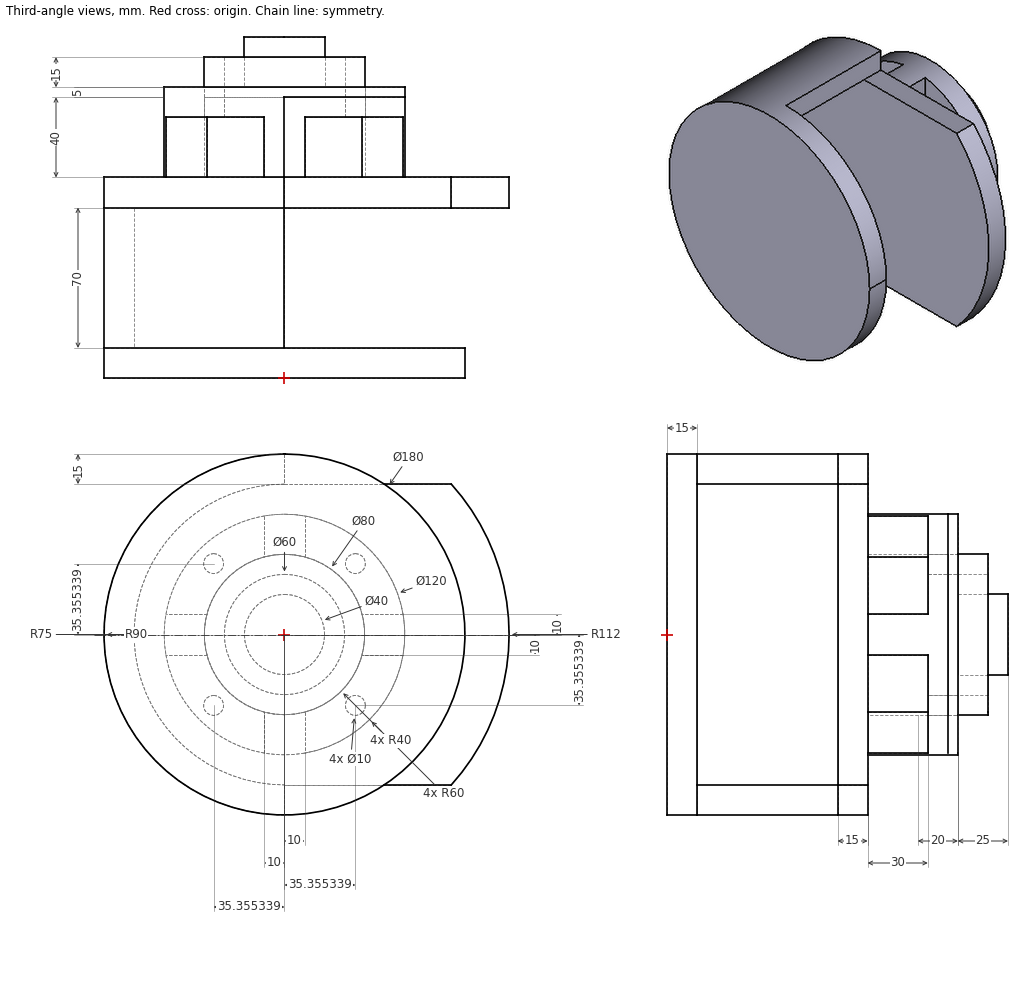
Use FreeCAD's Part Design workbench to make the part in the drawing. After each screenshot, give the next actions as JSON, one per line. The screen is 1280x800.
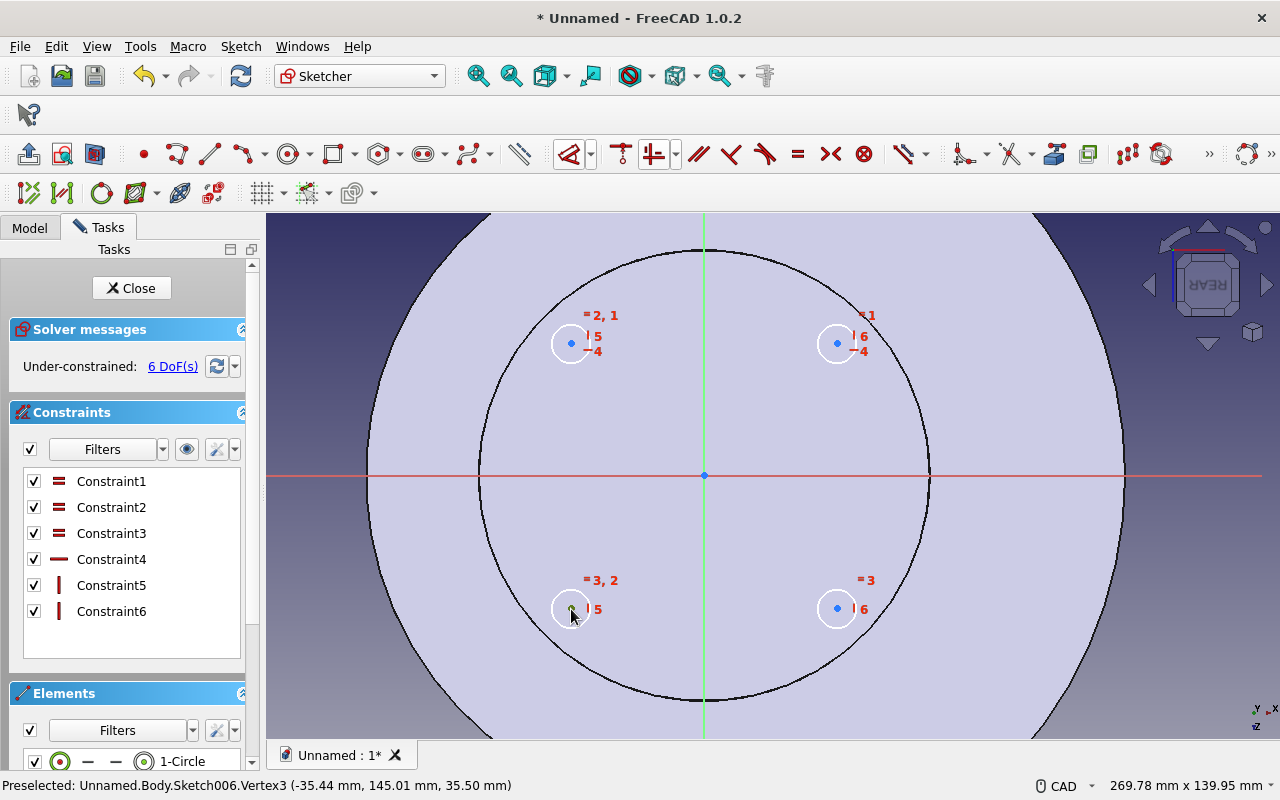
{"action": "left_click", "coordinate": [837, 609]}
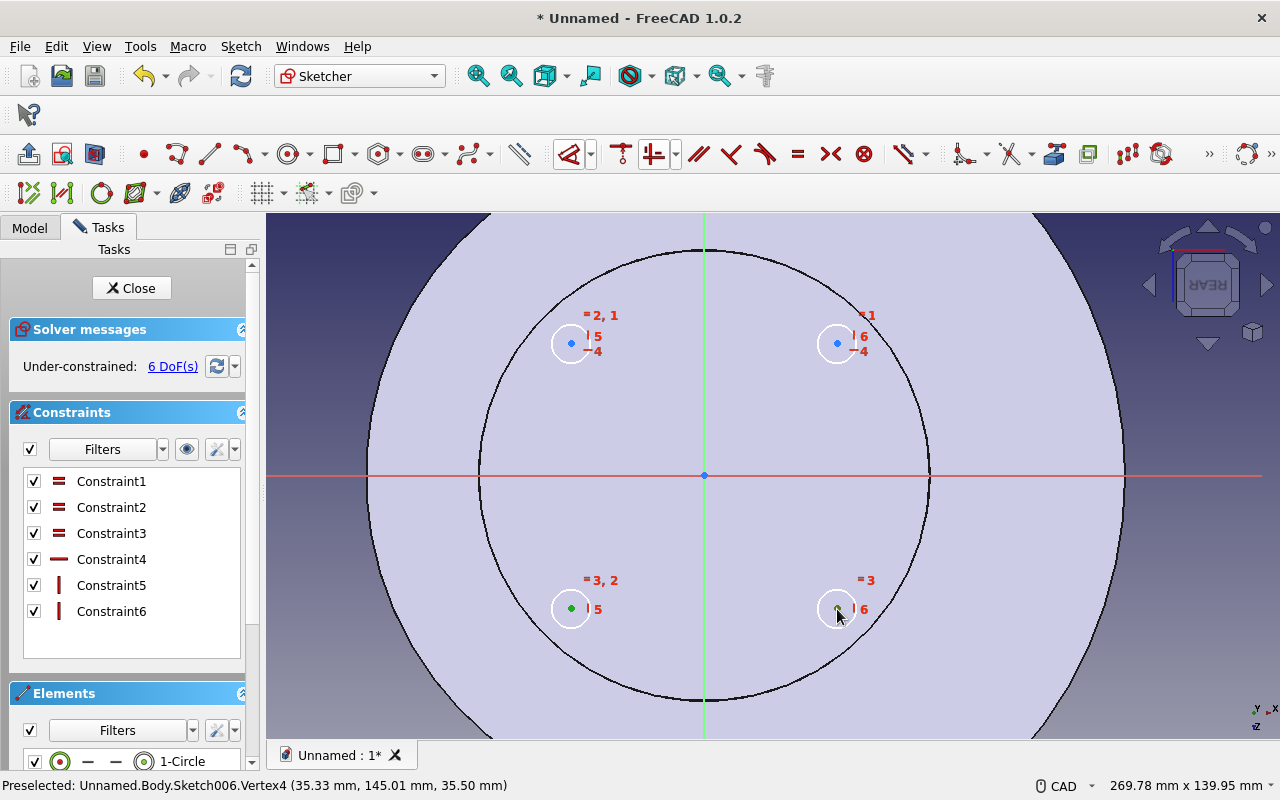
{"action": "left_click", "coordinate": [676, 154]}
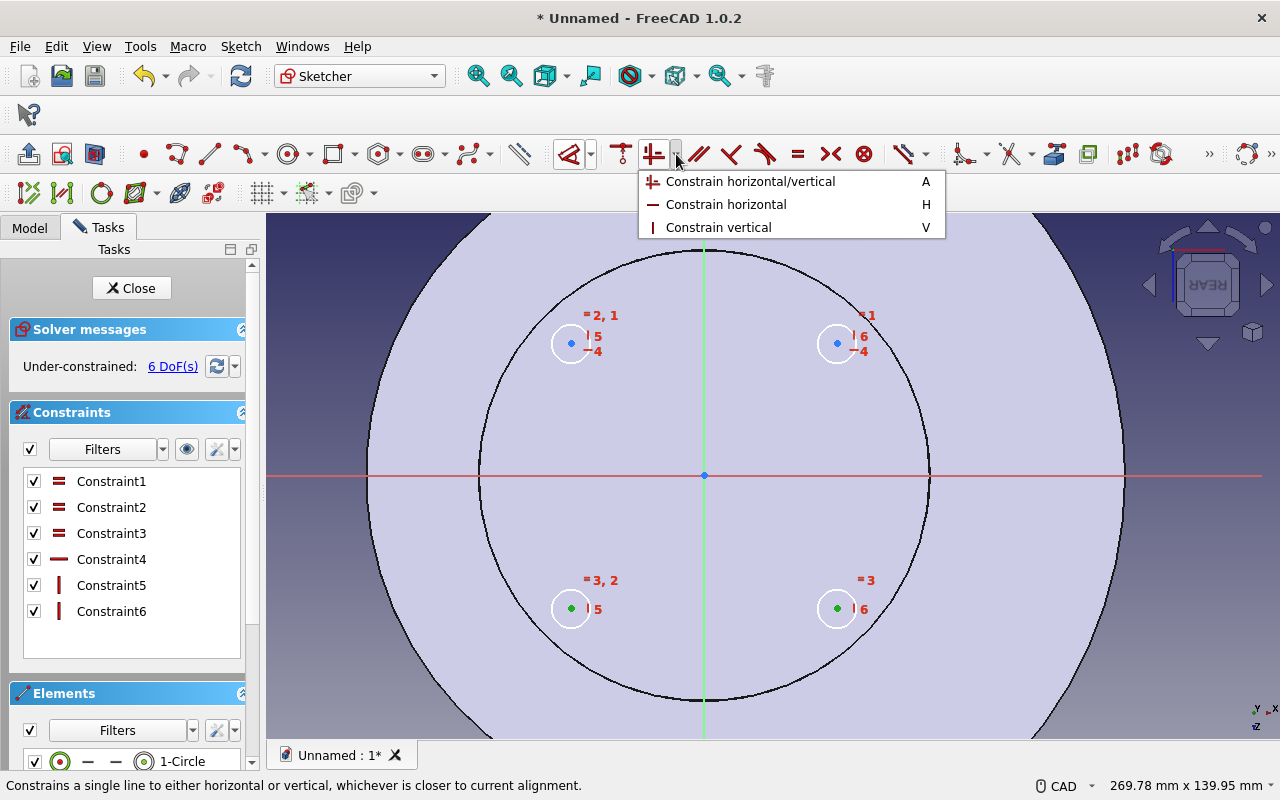
{"action": "left_click", "coordinate": [792, 204]}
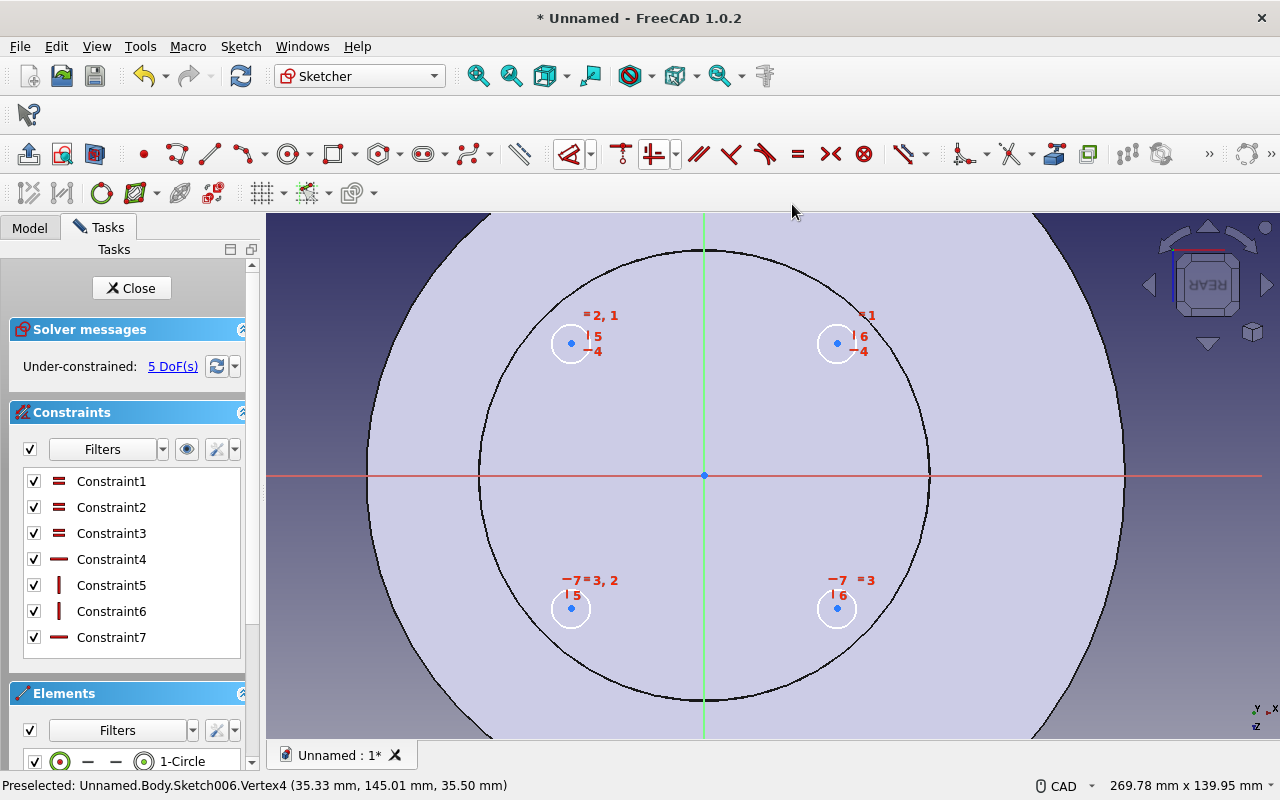
{"action": "left_click", "coordinate": [823, 331]}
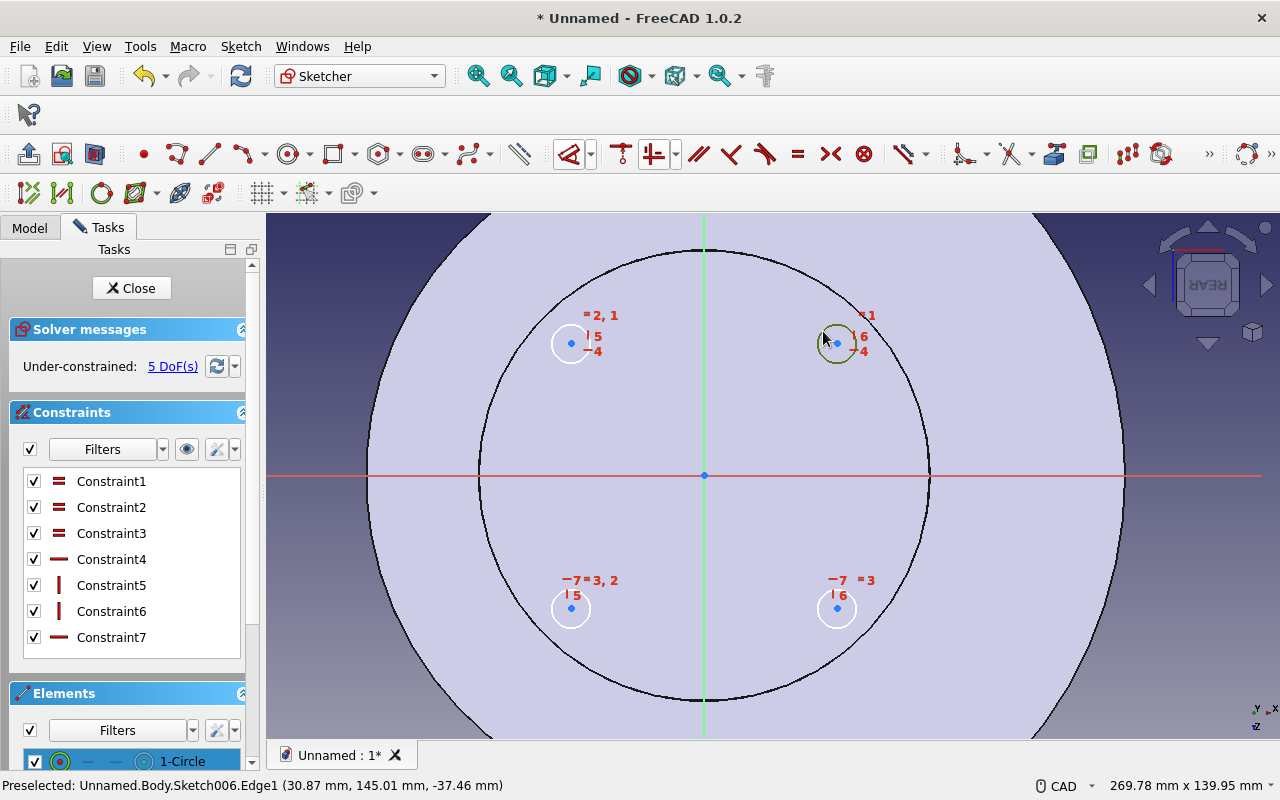
{"action": "key", "text": "k o"}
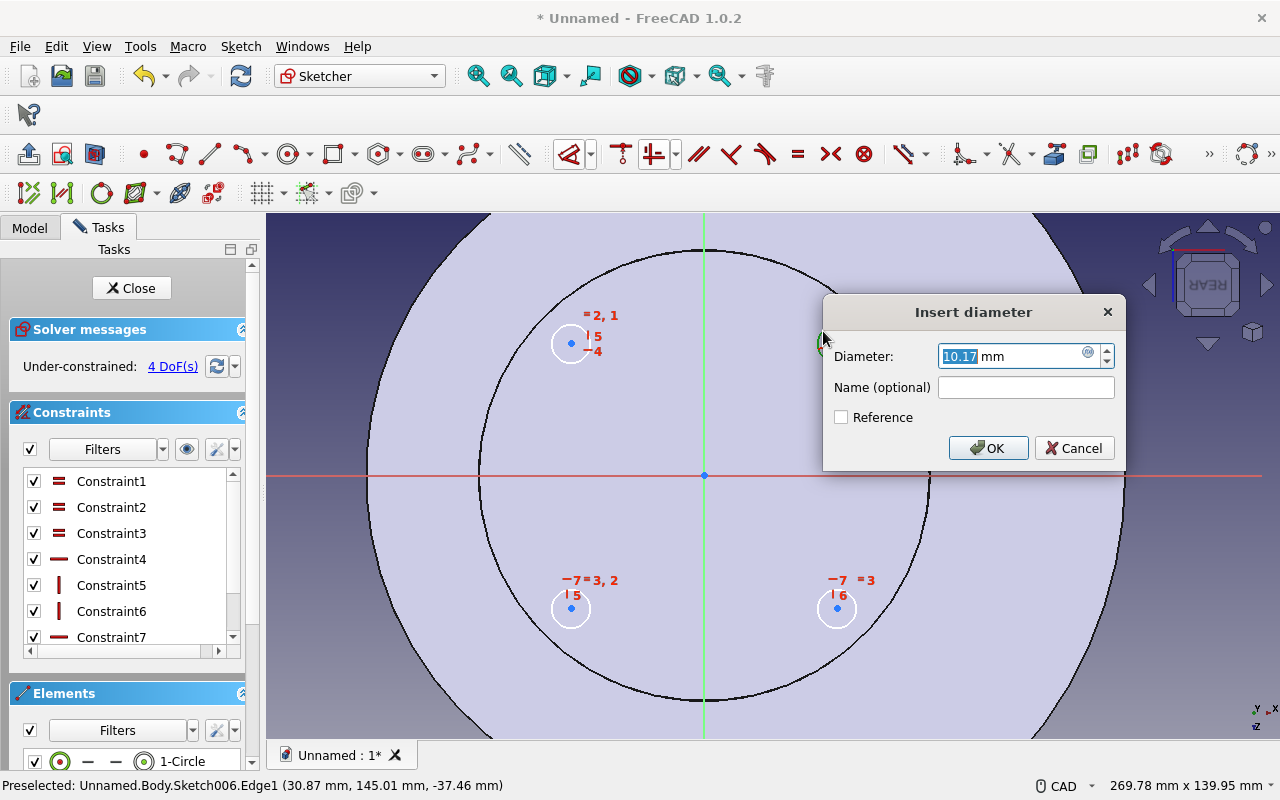
{"action": "type", "text": "10"}
{"action": "key", "text": "Return"}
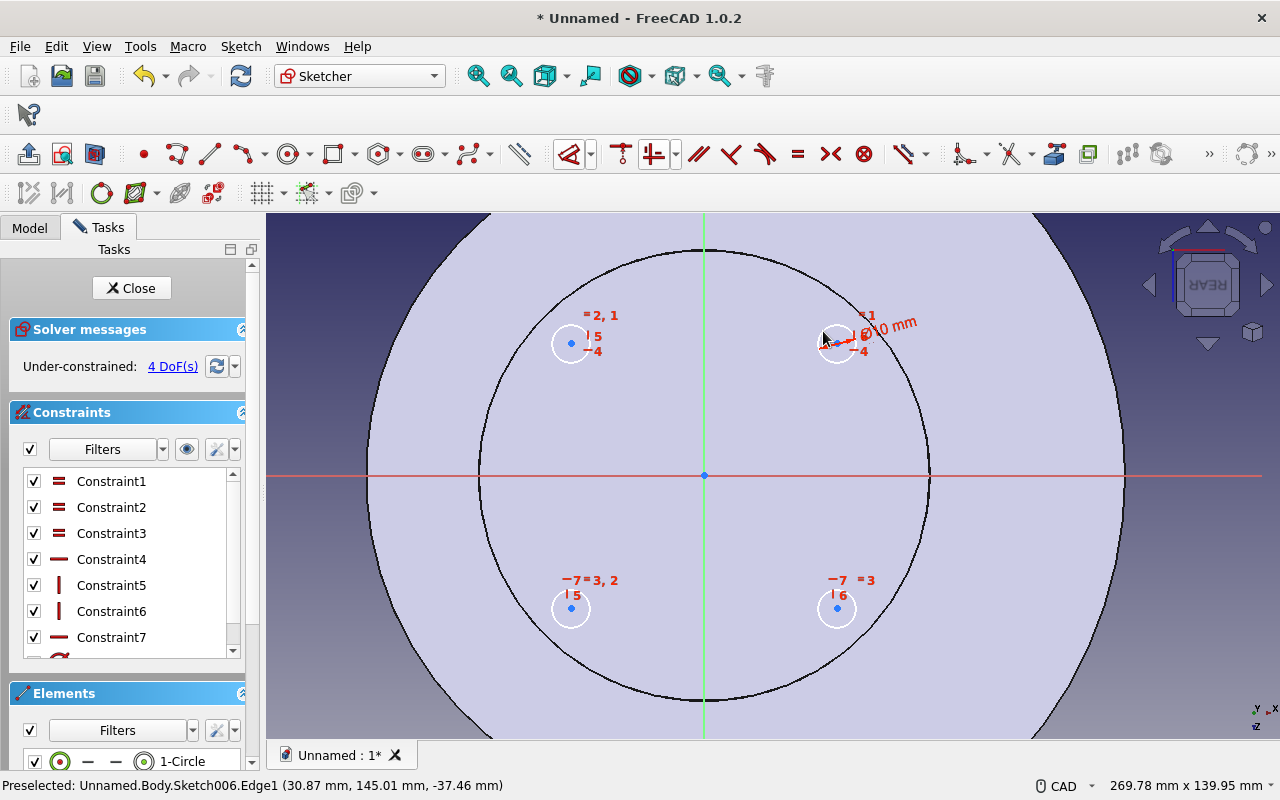
{"action": "left_click", "coordinate": [837, 344]}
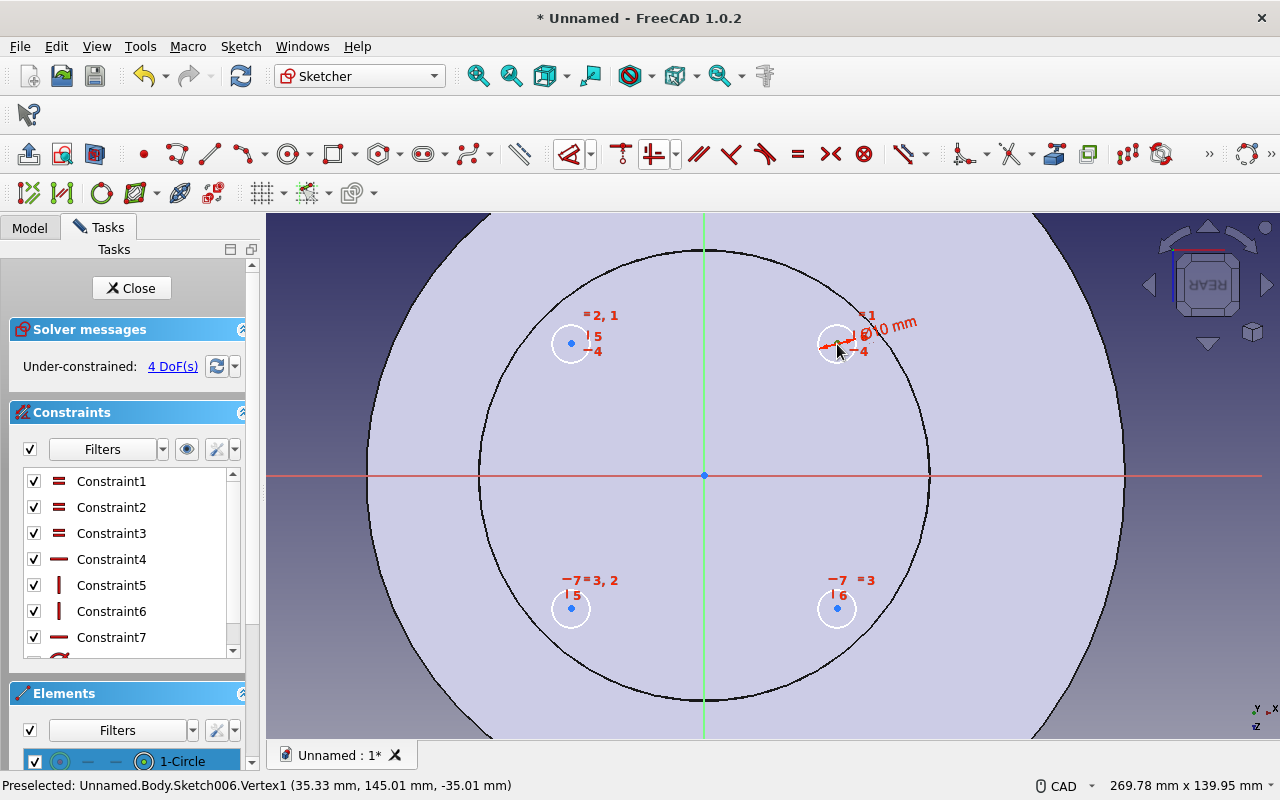
{"action": "key", "text": "l"}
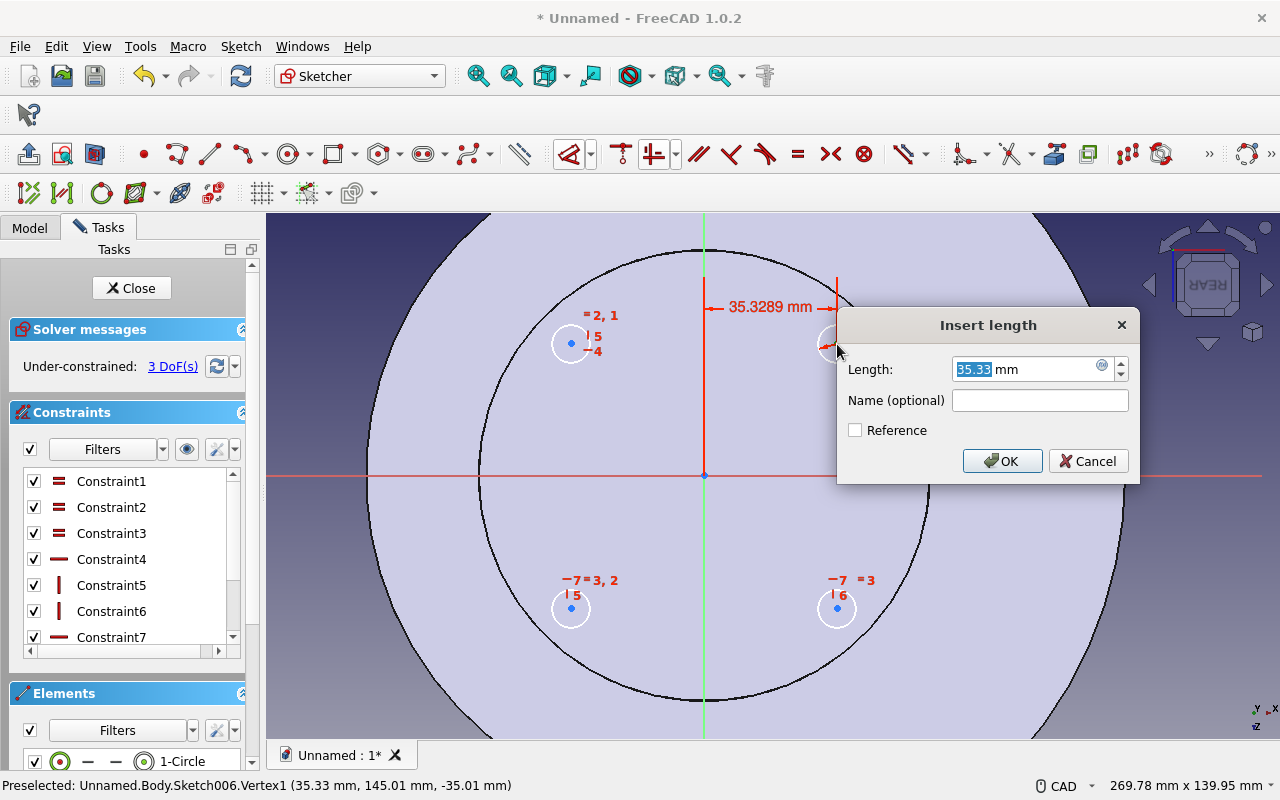
{"action": "type", "text": "35.355339"}
{"action": "key", "text": "Return"}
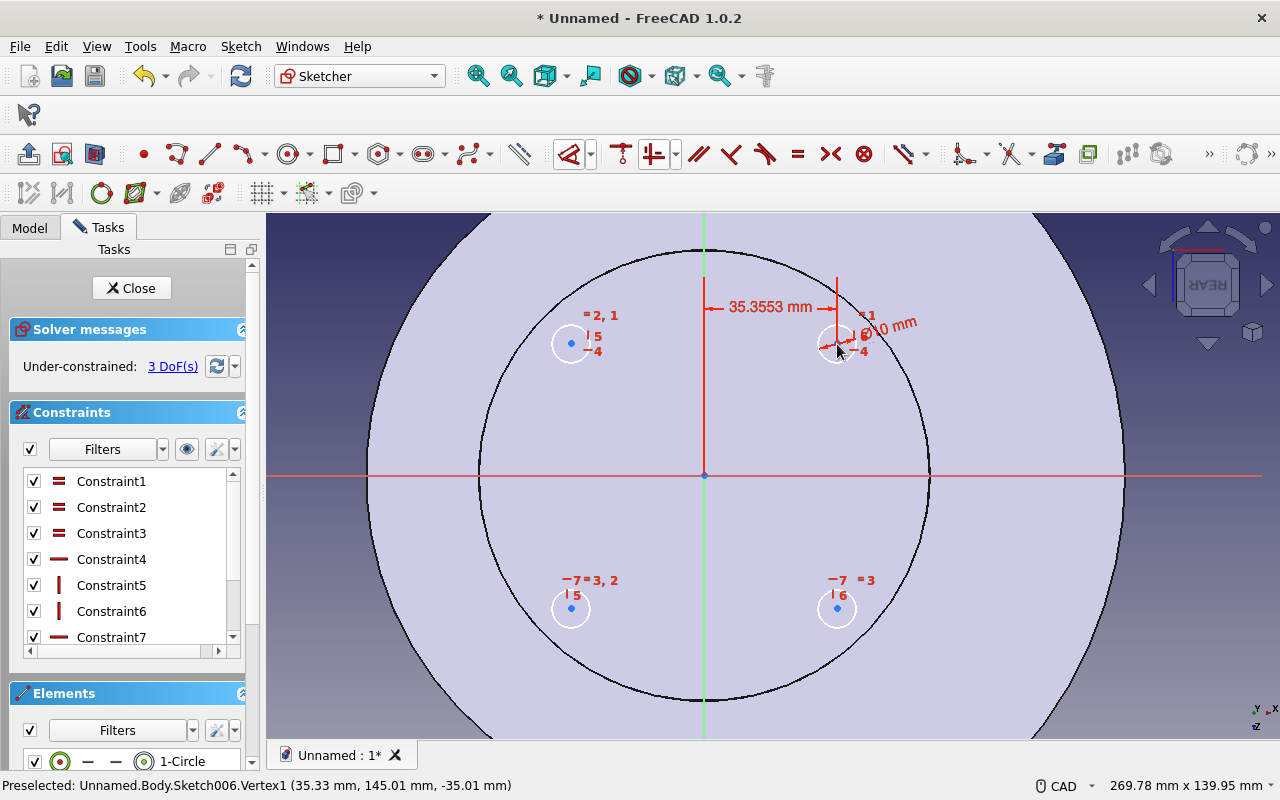
{"action": "left_click", "coordinate": [837, 344]}